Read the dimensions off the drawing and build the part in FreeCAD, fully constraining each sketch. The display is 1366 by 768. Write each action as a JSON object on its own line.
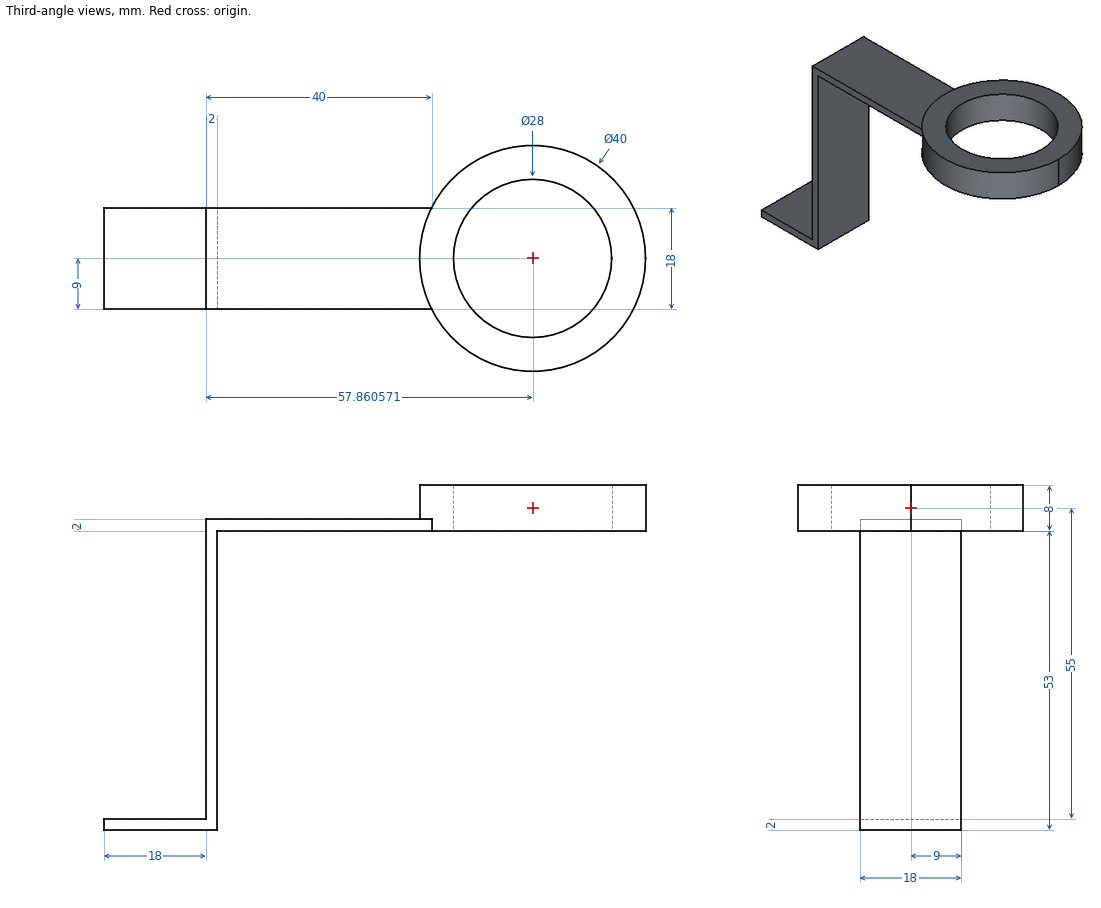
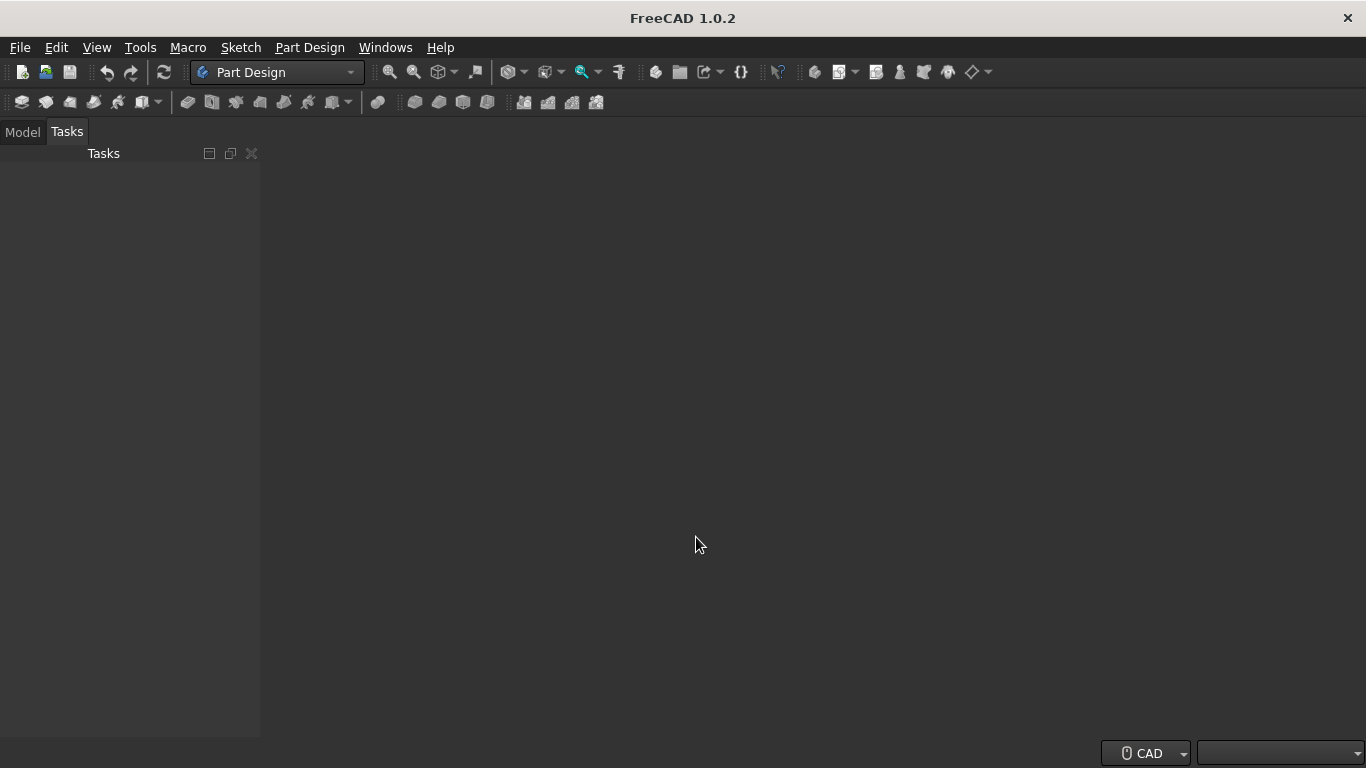
{"action": "left_click", "coordinate": [22, 72]}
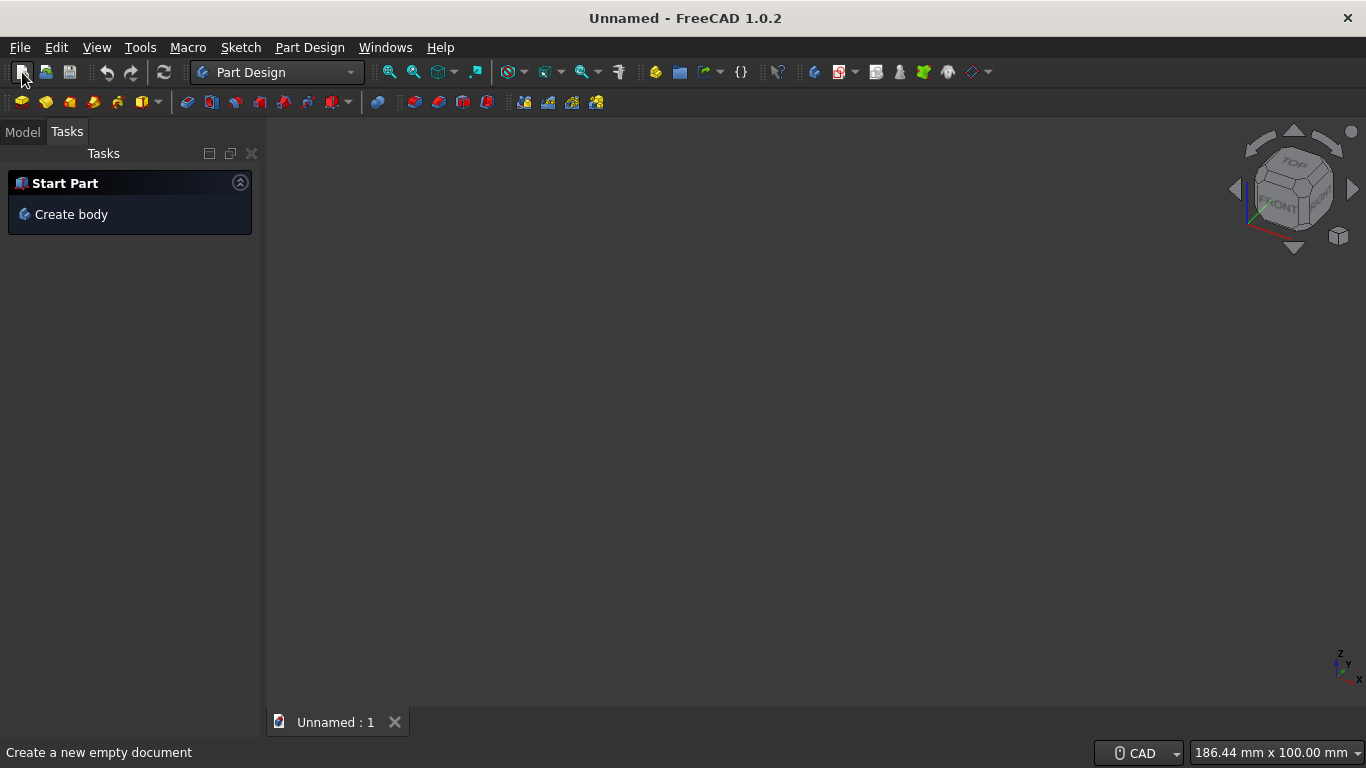
{"action": "left_click", "coordinate": [840, 72]}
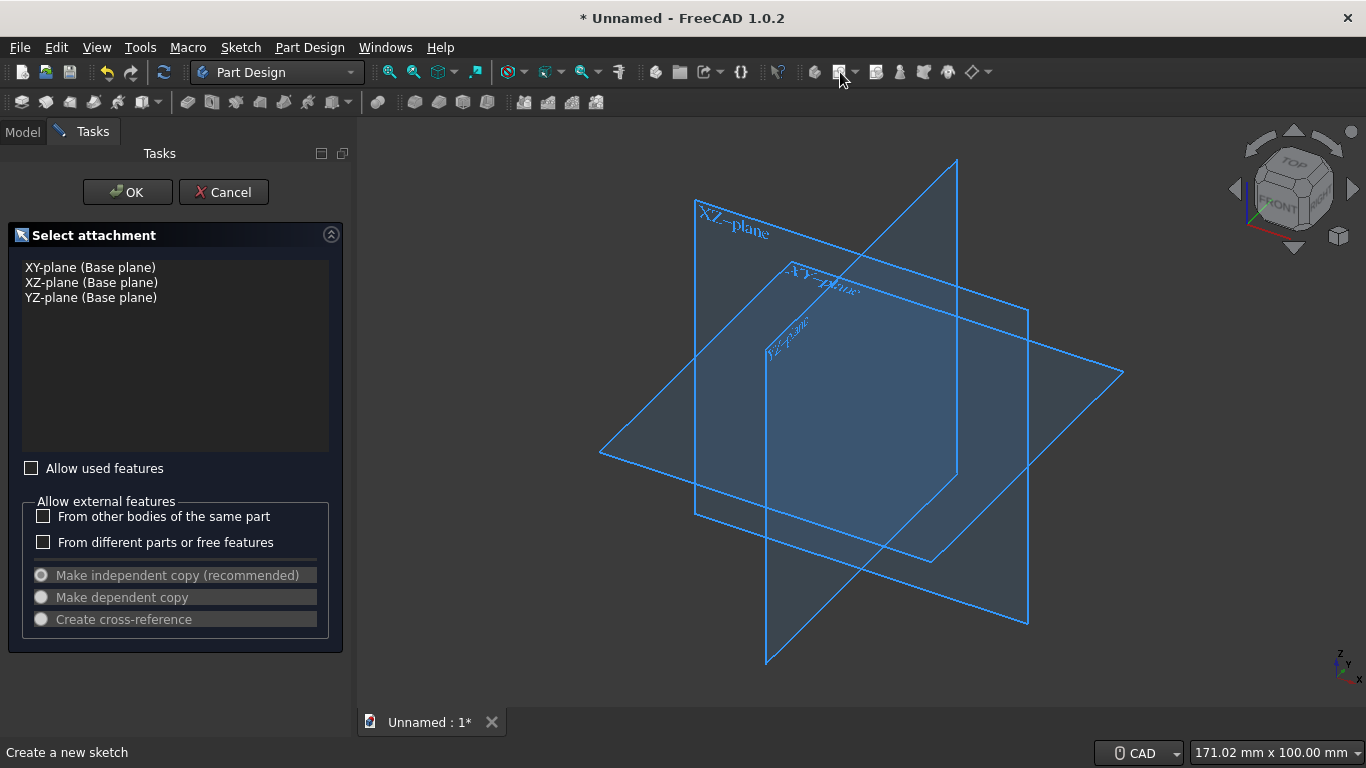
{"action": "left_click", "coordinate": [82, 268]}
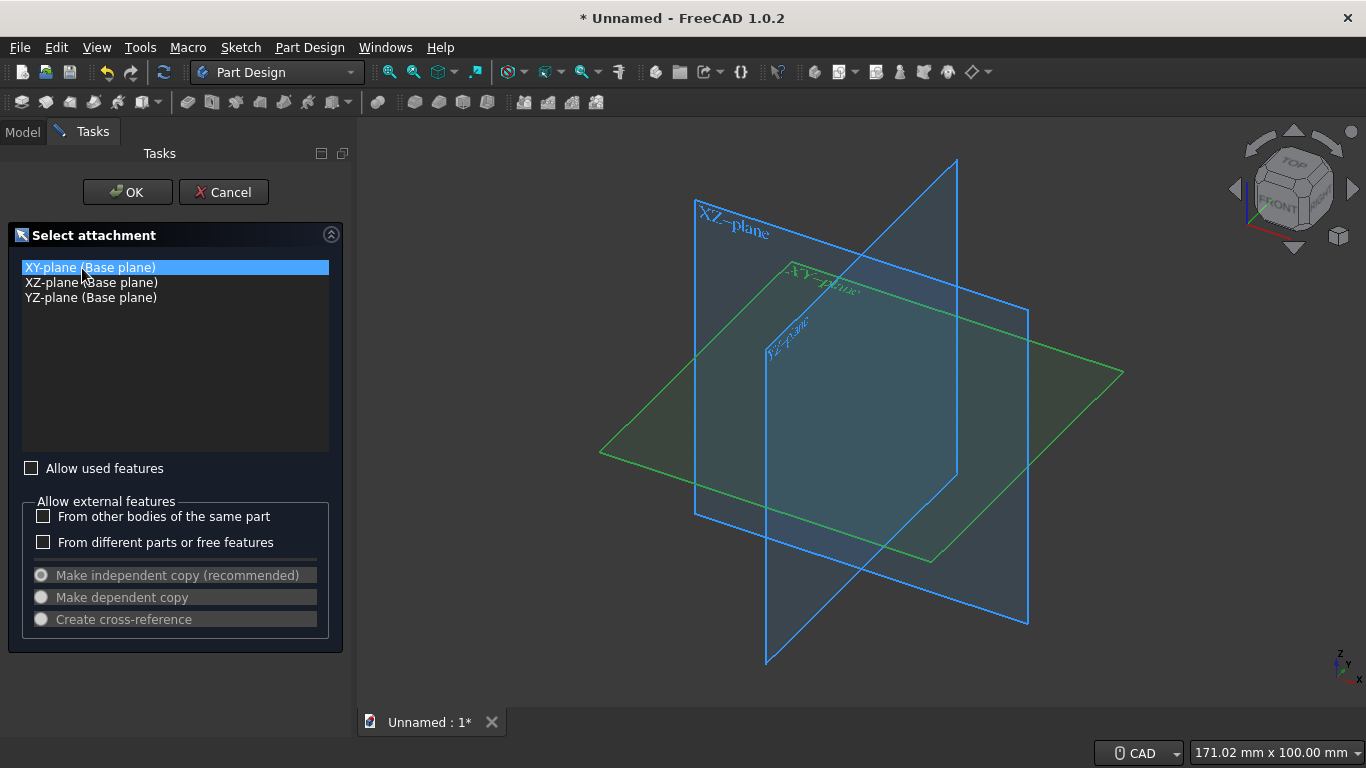
{"action": "left_click", "coordinate": [128, 192]}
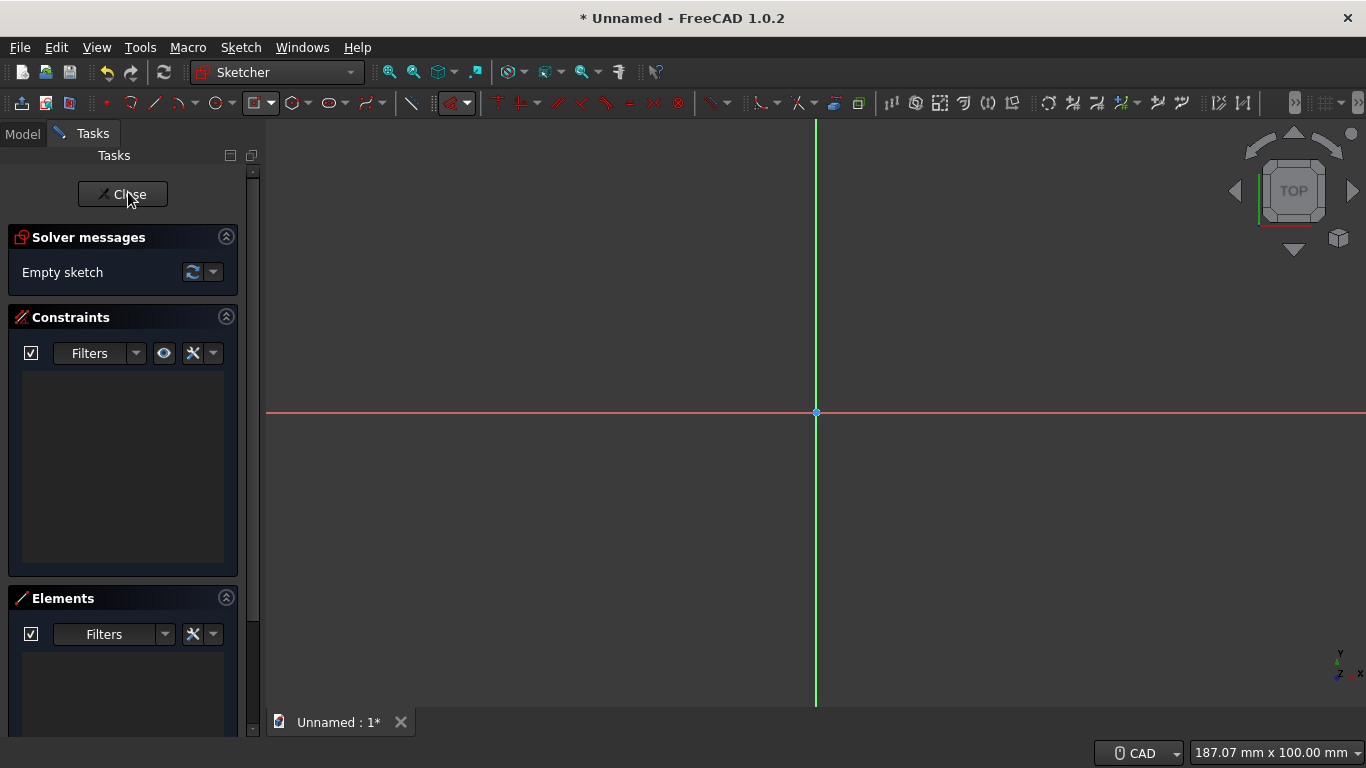
{"action": "scroll", "coordinate": [955, 413], "scroll_direction": "up", "scroll_amount": 2}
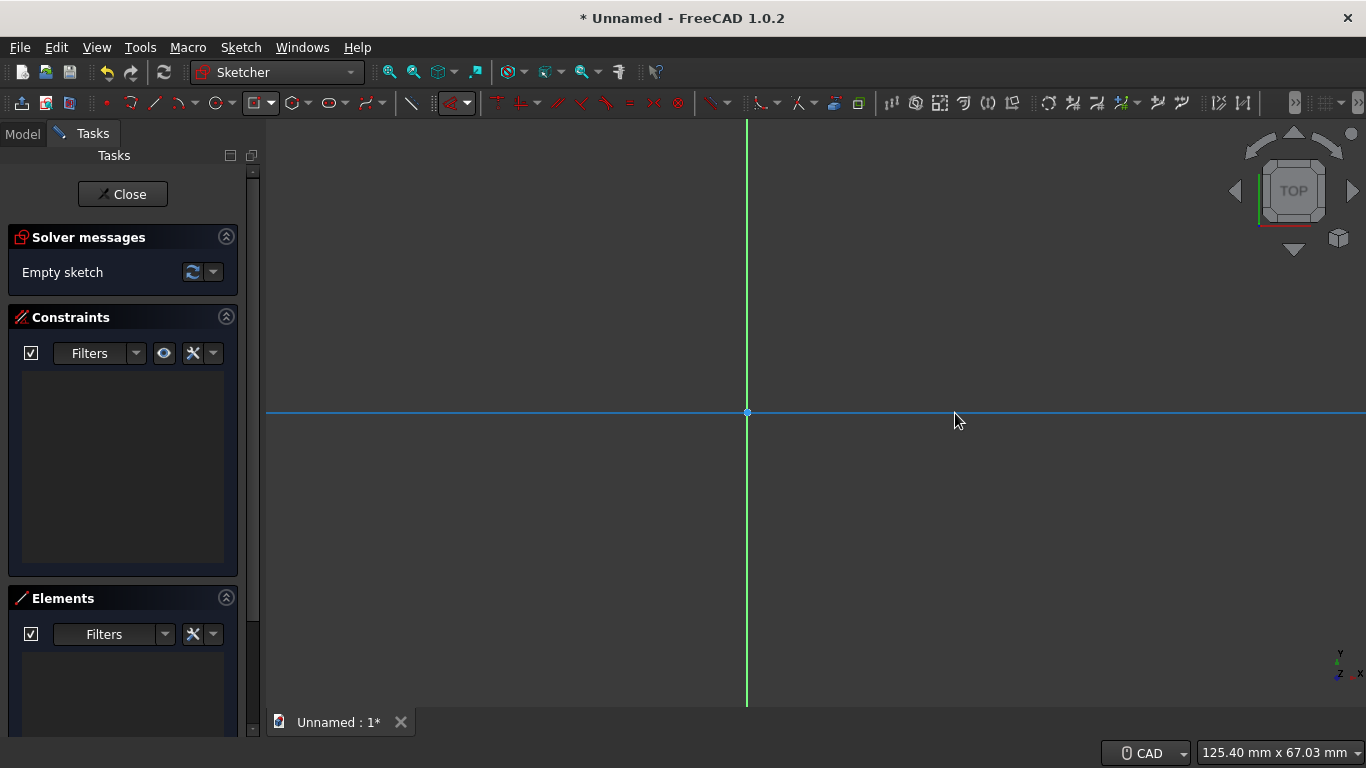
{"action": "left_click", "coordinate": [216, 104]}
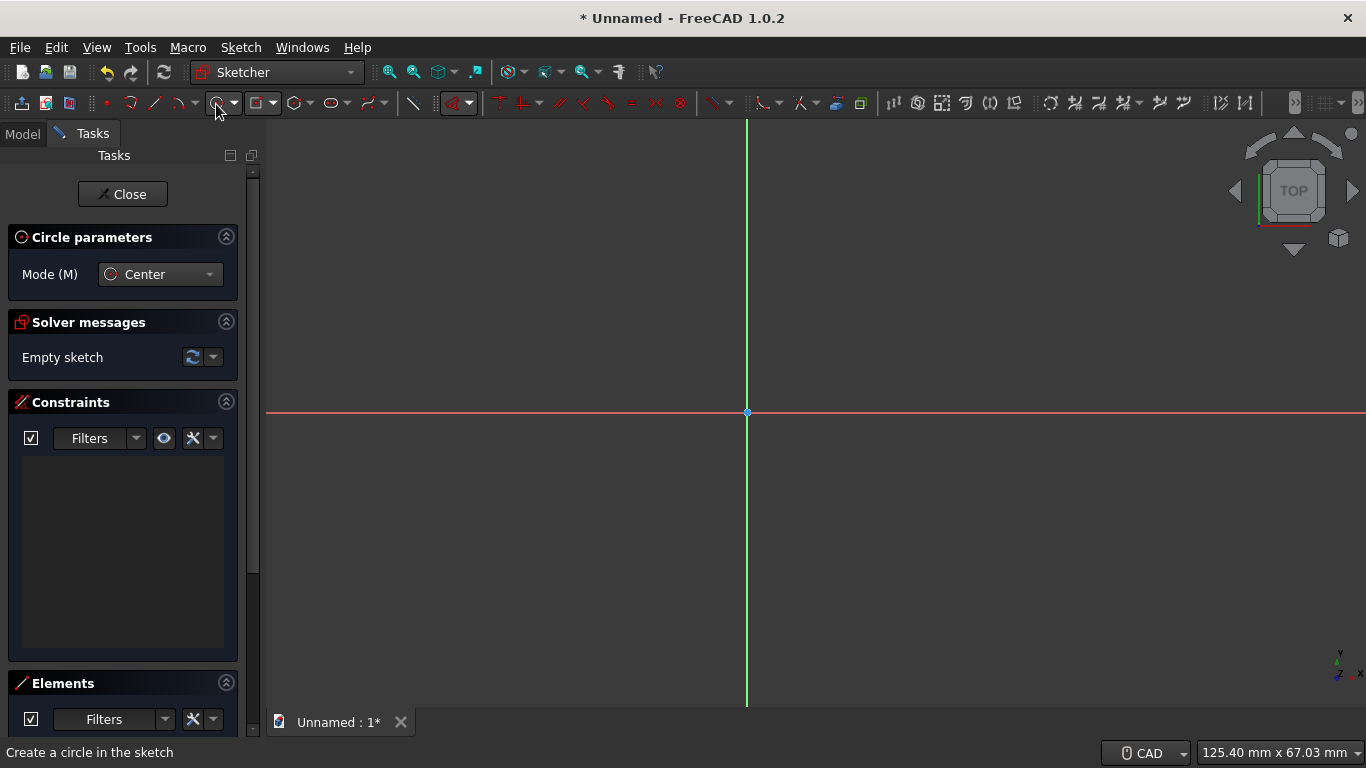
{"action": "left_click", "coordinate": [747, 413]}
{"action": "mouse_move", "coordinate": [871, 289]}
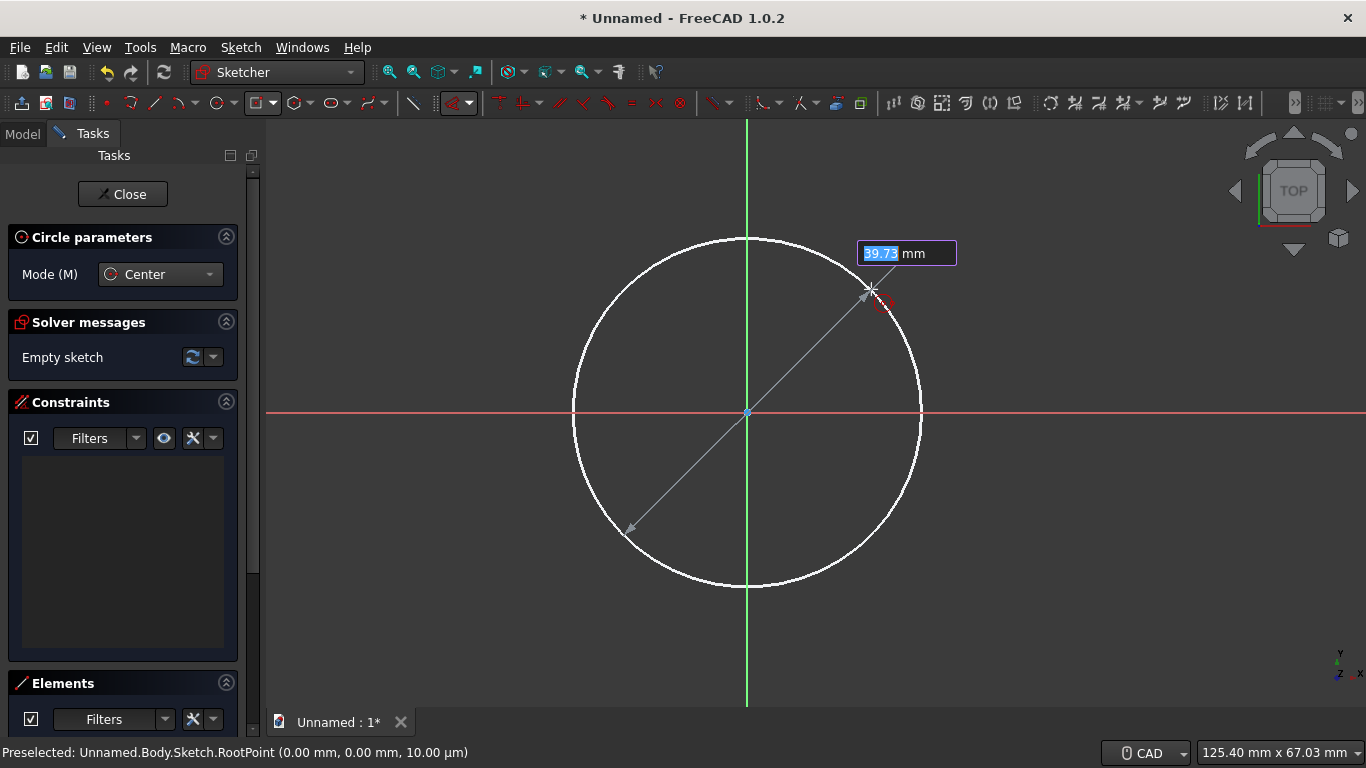
{"action": "type", "text": "40"}
{"action": "key", "text": "Return"}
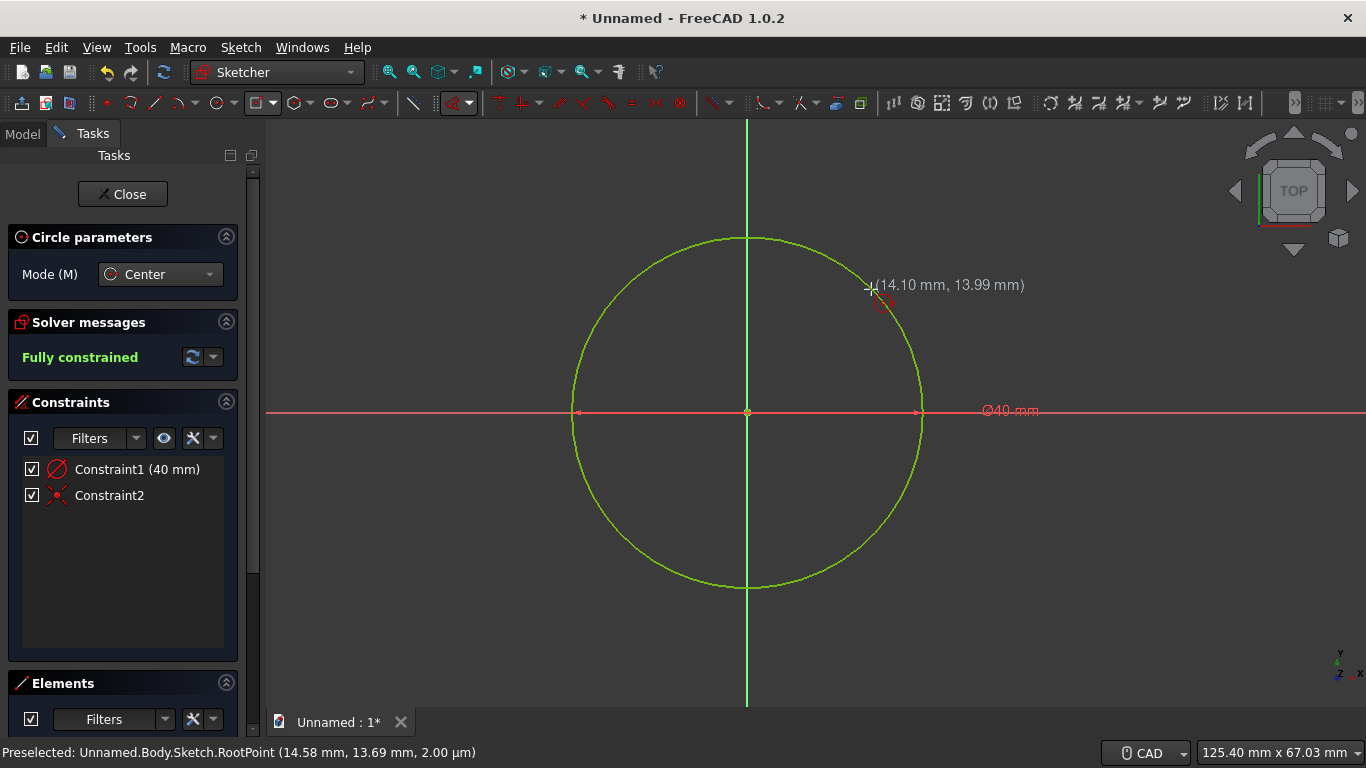
{"action": "left_click", "coordinate": [747, 413]}
{"action": "mouse_move", "coordinate": [834, 326]}